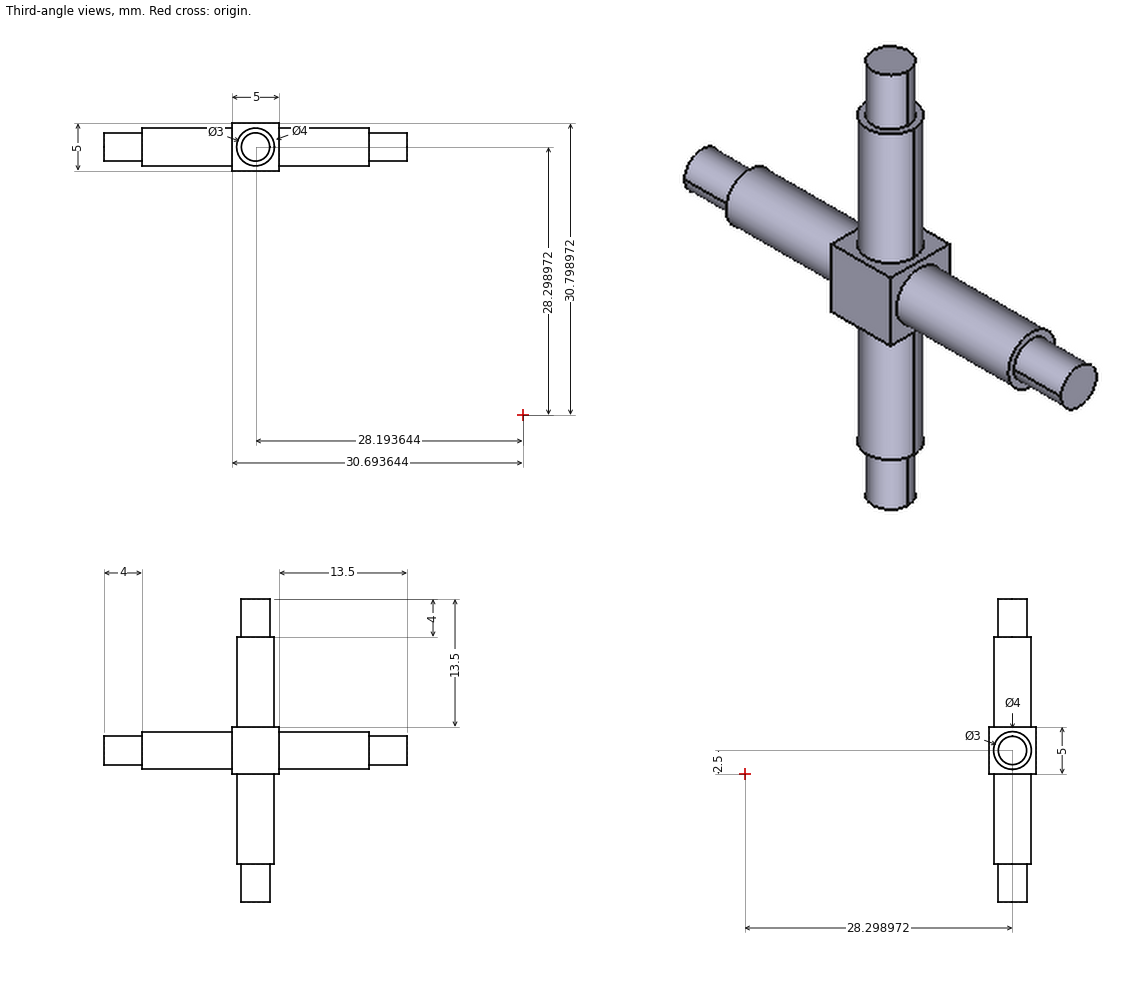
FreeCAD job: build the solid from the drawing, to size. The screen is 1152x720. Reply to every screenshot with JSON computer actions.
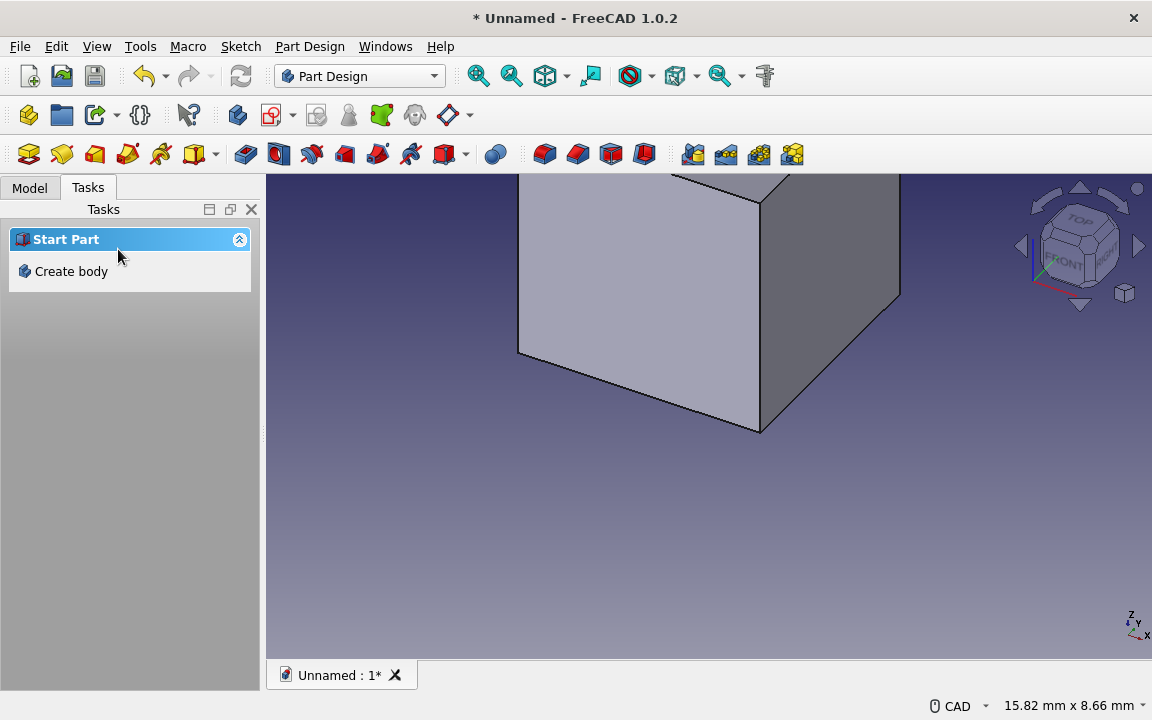
{"action": "key", "text": "v f"}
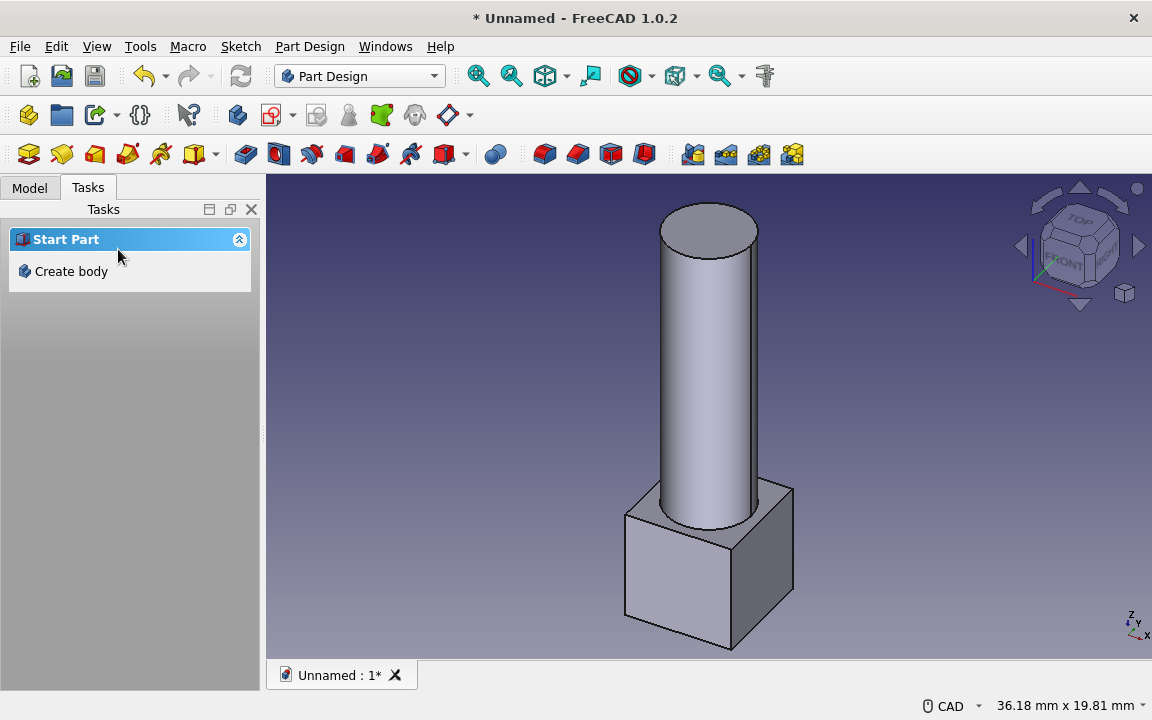
{"action": "left_click", "coordinate": [762, 568]}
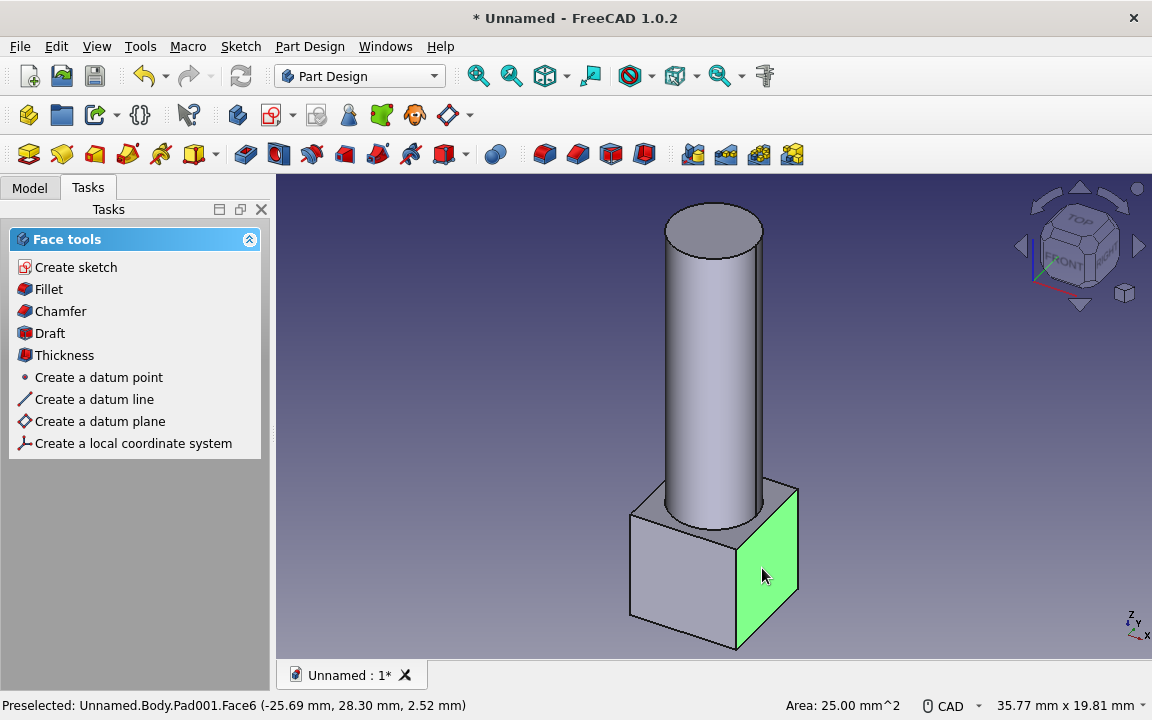
{"action": "left_click", "coordinate": [270, 116]}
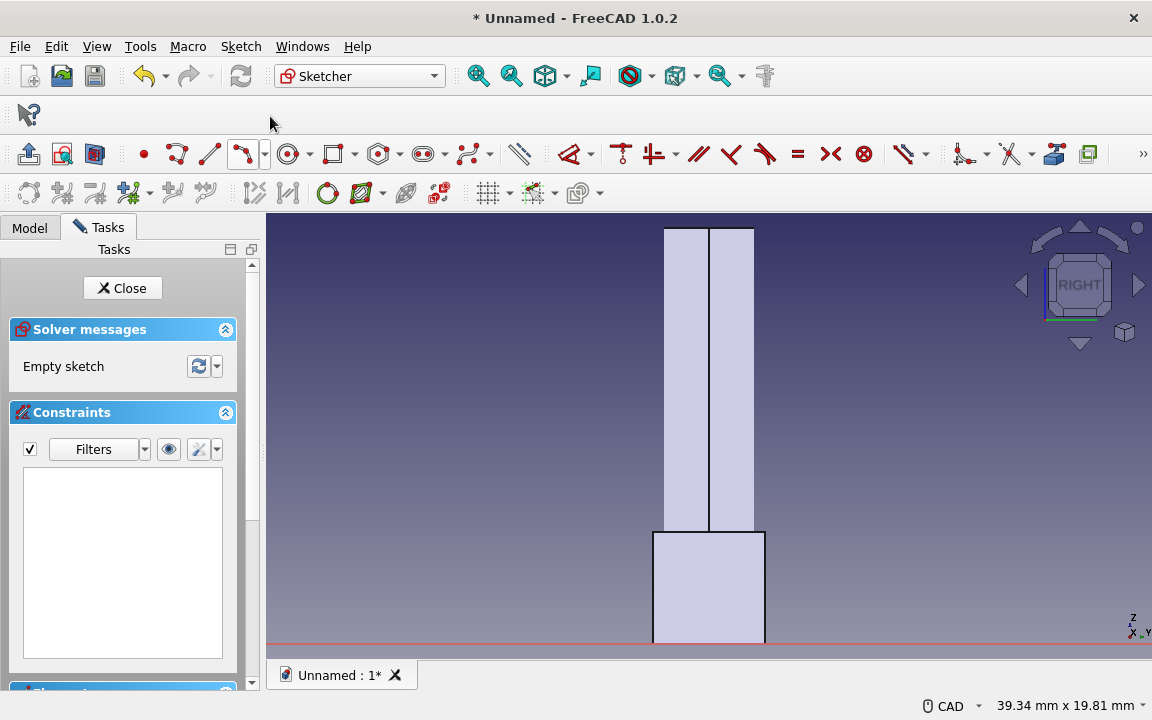
{"action": "scroll", "coordinate": [640, 436], "scroll_direction": "down", "scroll_amount": 5}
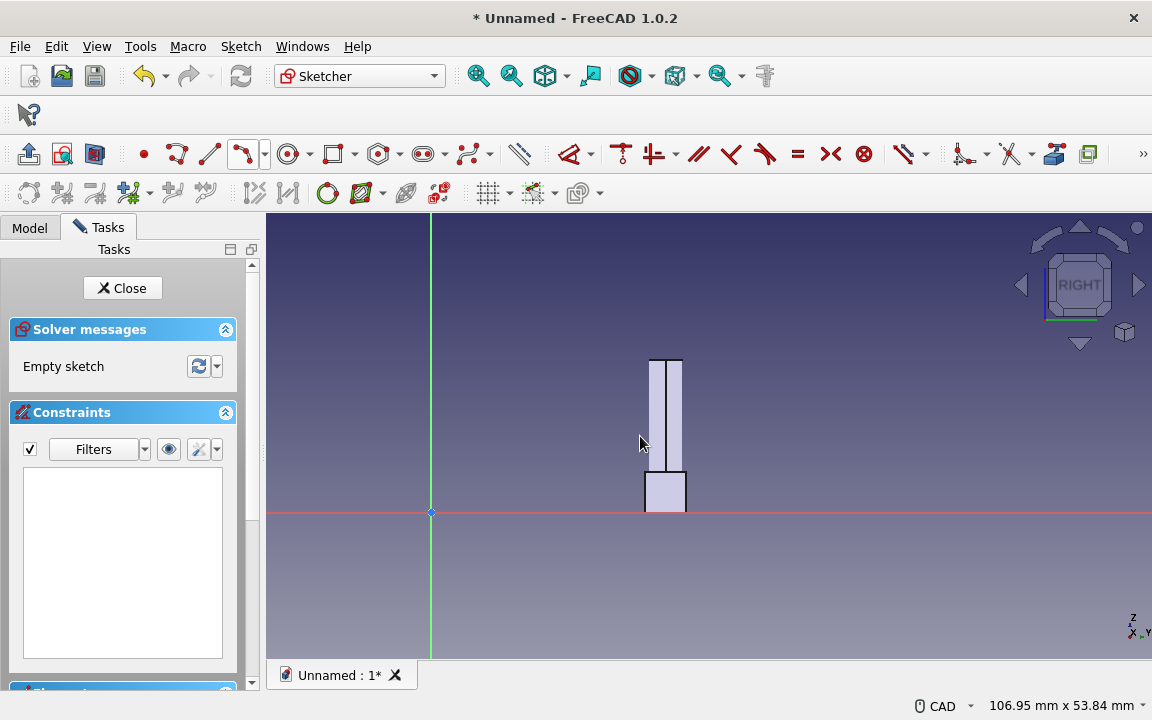
{"action": "scroll", "coordinate": [669, 499], "scroll_direction": "up", "scroll_amount": 11}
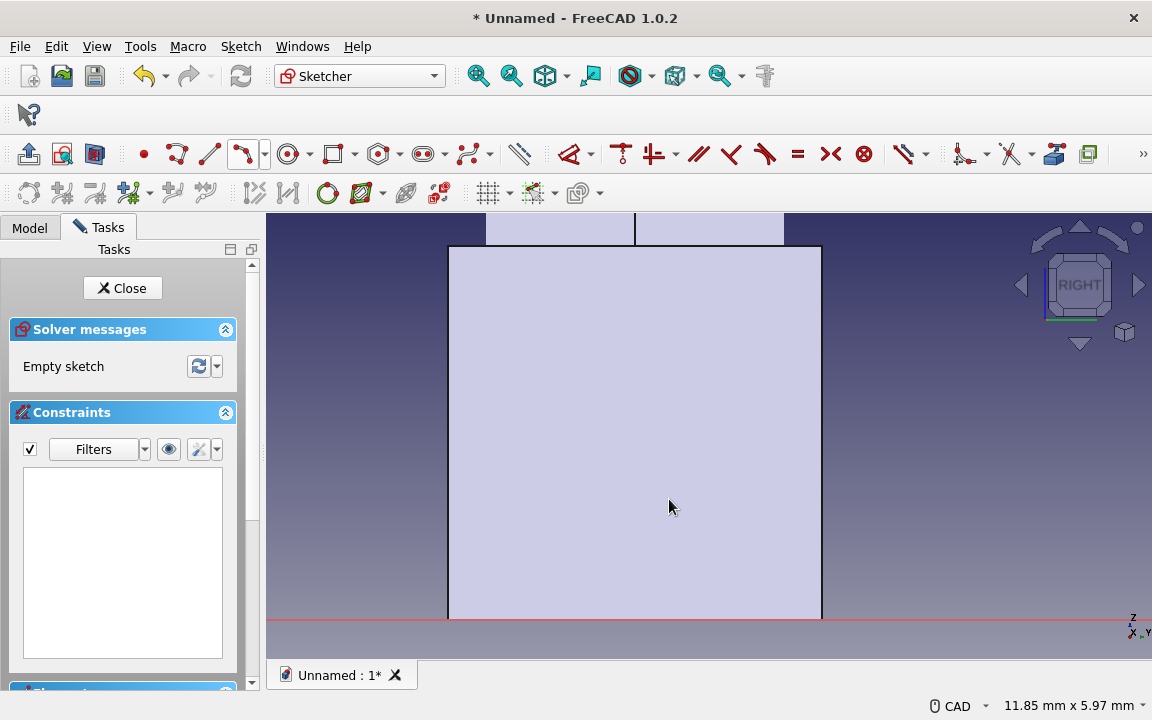
{"action": "left_click", "coordinate": [288, 154]}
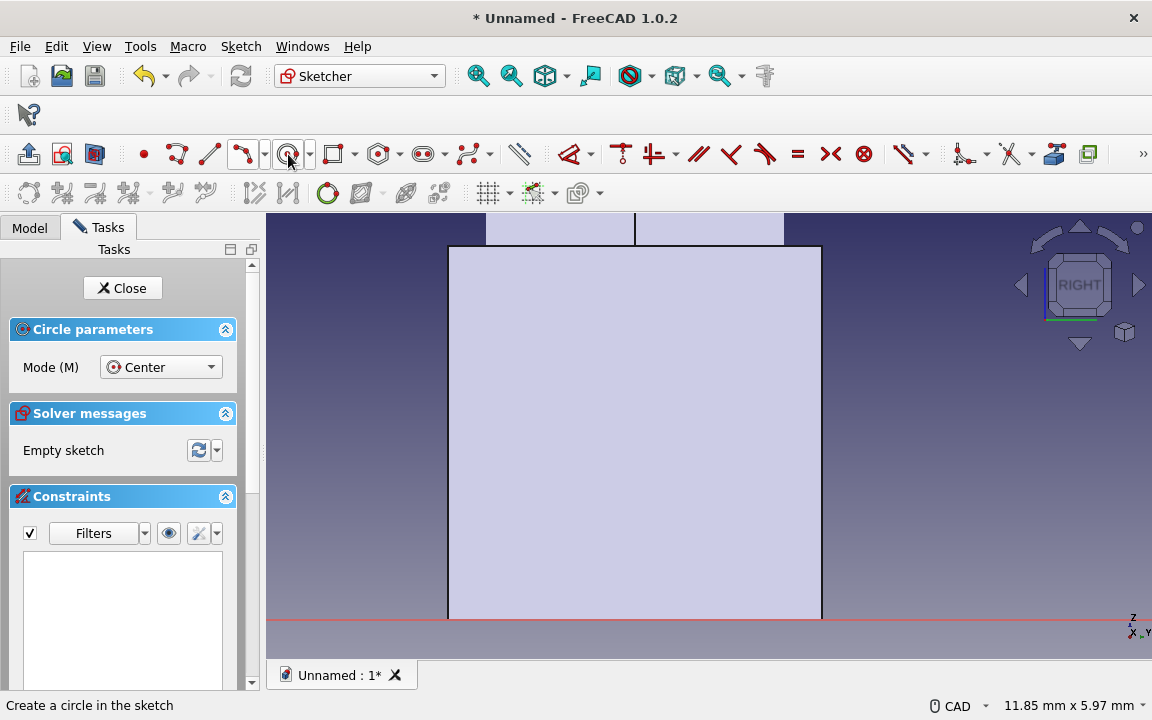
{"action": "left_click", "coordinate": [635, 433]}
{"action": "left_click", "coordinate": [741, 327]}
{"action": "key", "text": "Escape"}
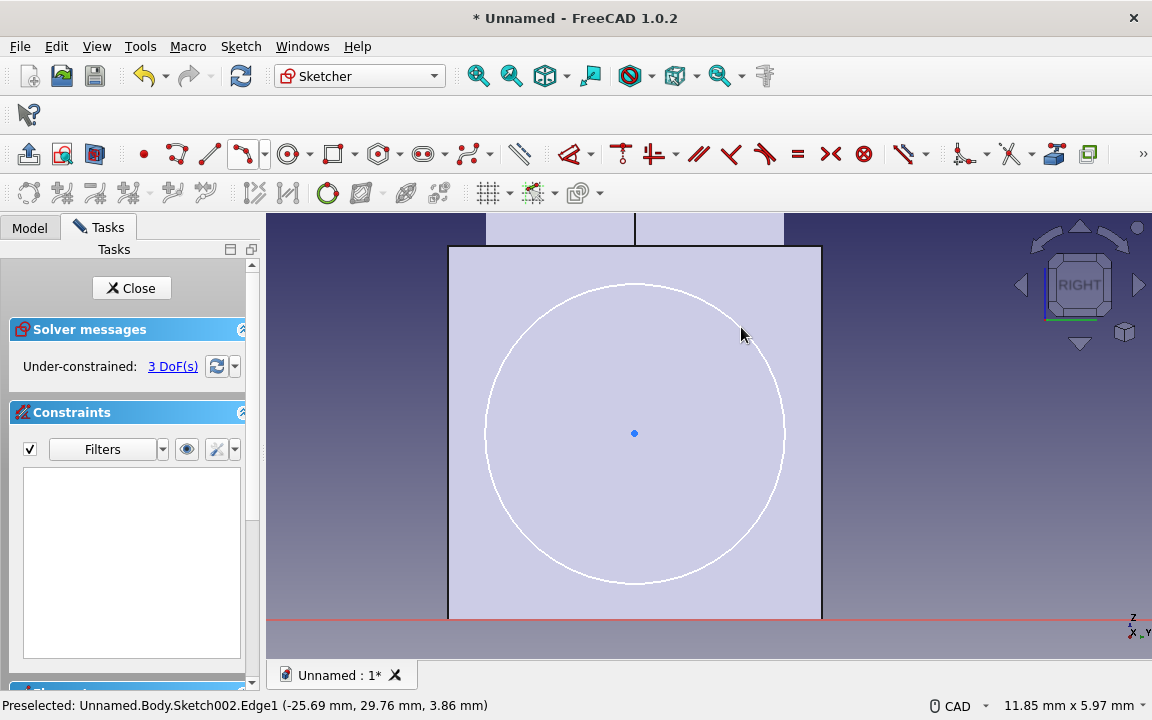
{"action": "key", "text": "d"}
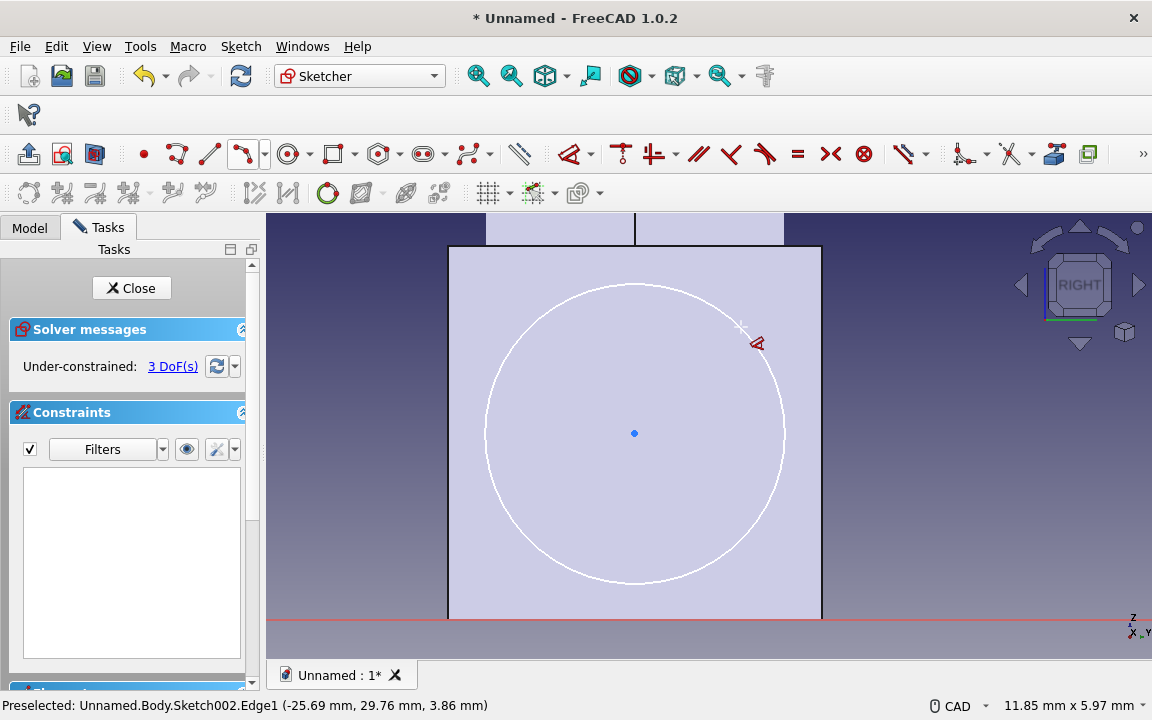
{"action": "left_click", "coordinate": [741, 328]}
{"action": "left_click", "coordinate": [764, 305]}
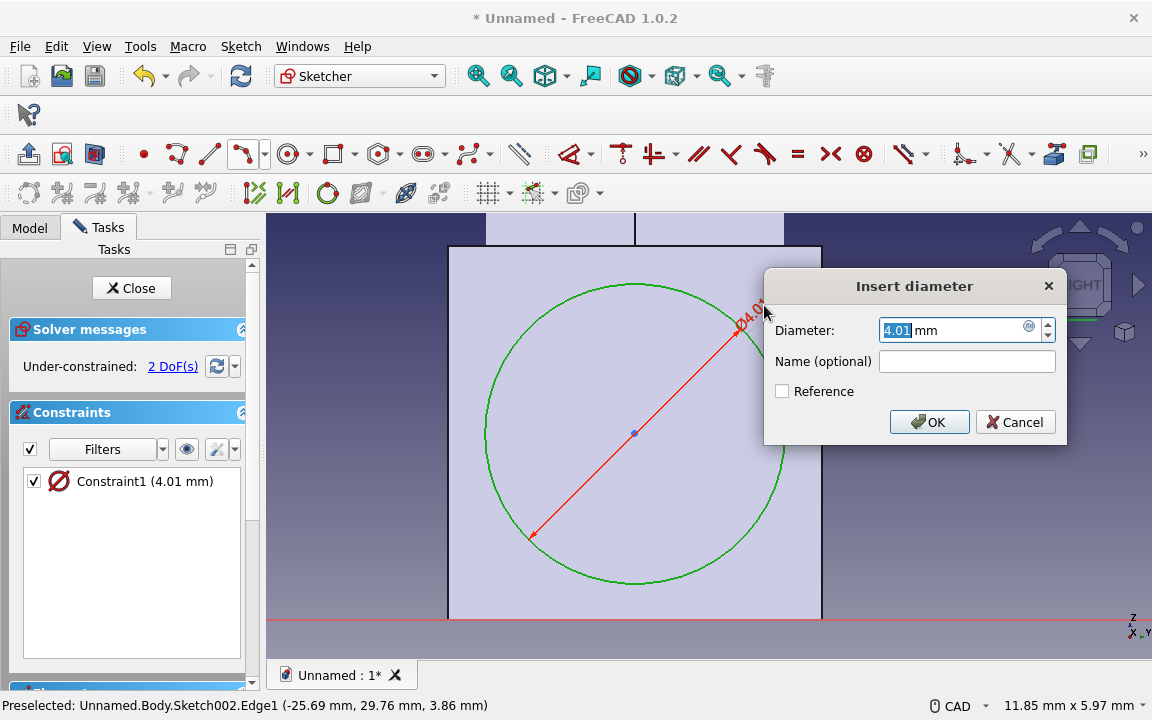
{"action": "type", "text": "4"}
{"action": "key", "text": "Return"}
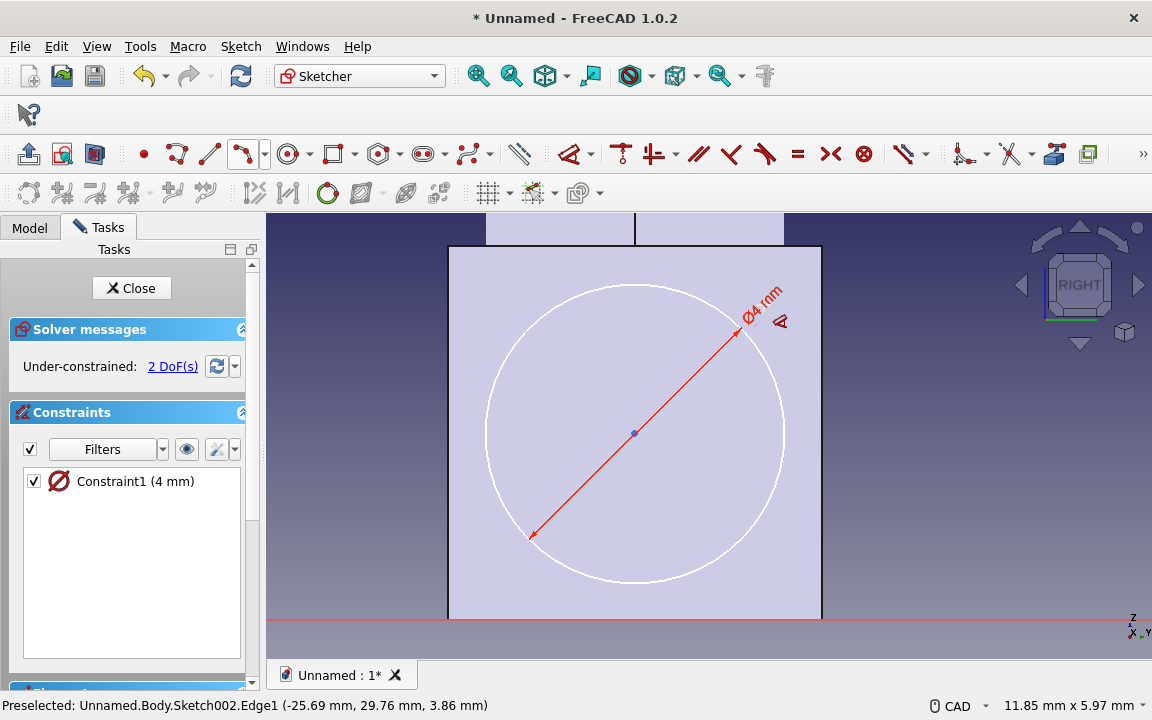
{"action": "left_click", "coordinate": [635, 434]}
{"action": "left_click", "coordinate": [669, 527]}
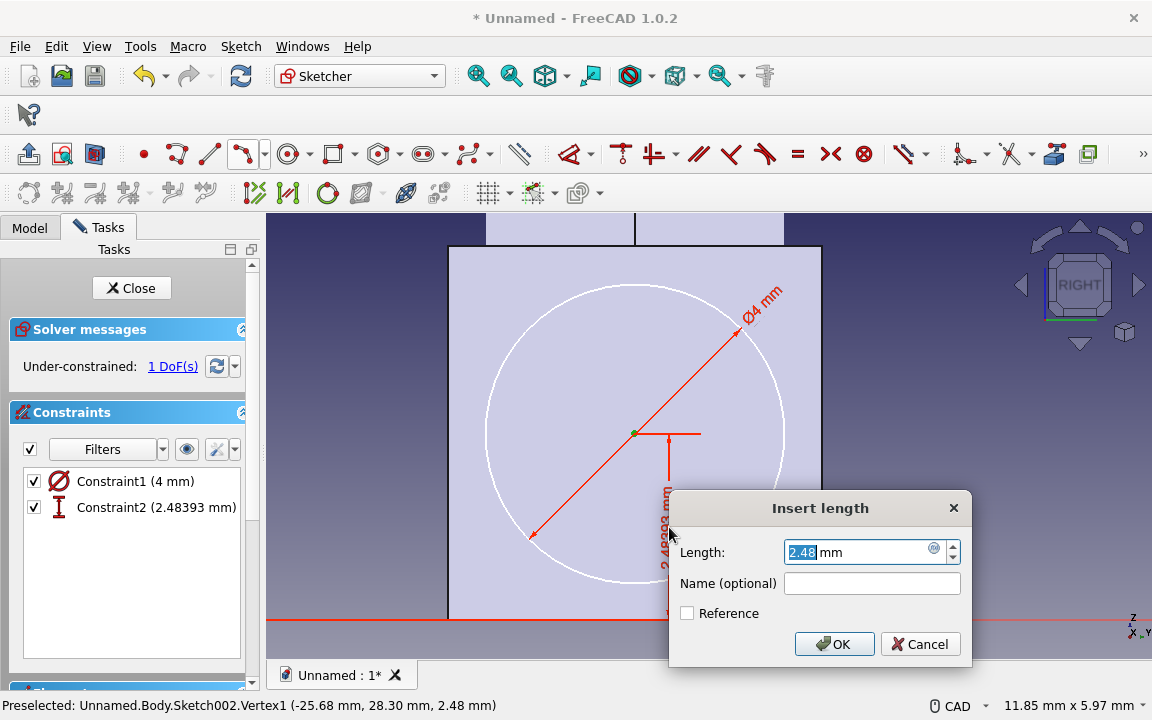
{"action": "type", "text": "2.5"}
{"action": "key", "text": "Return"}